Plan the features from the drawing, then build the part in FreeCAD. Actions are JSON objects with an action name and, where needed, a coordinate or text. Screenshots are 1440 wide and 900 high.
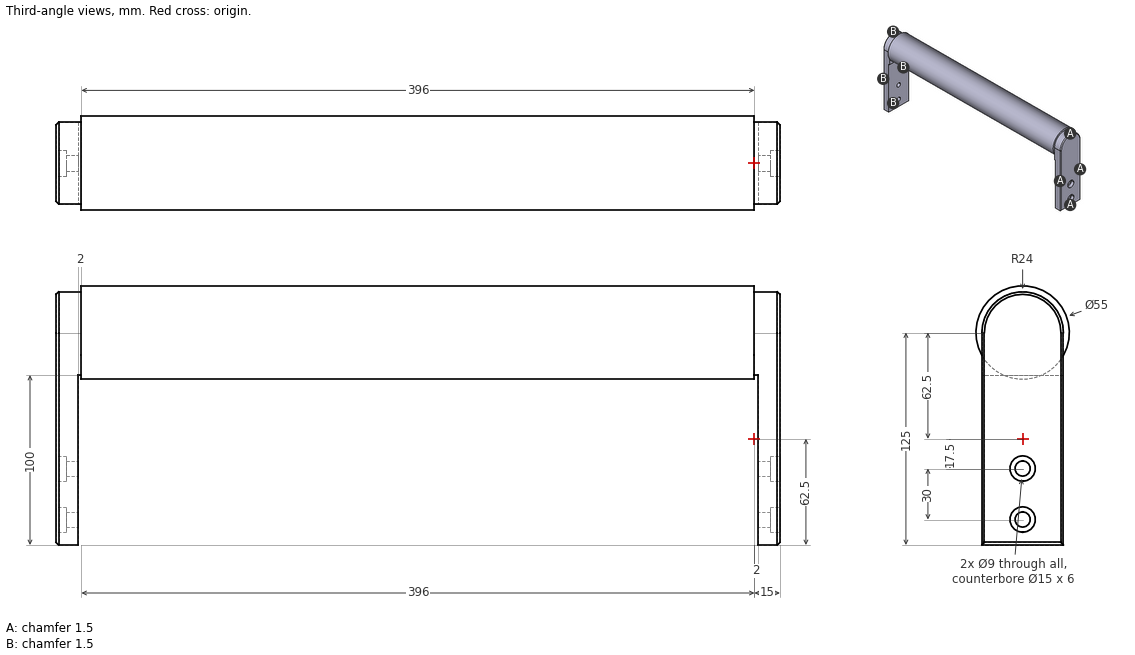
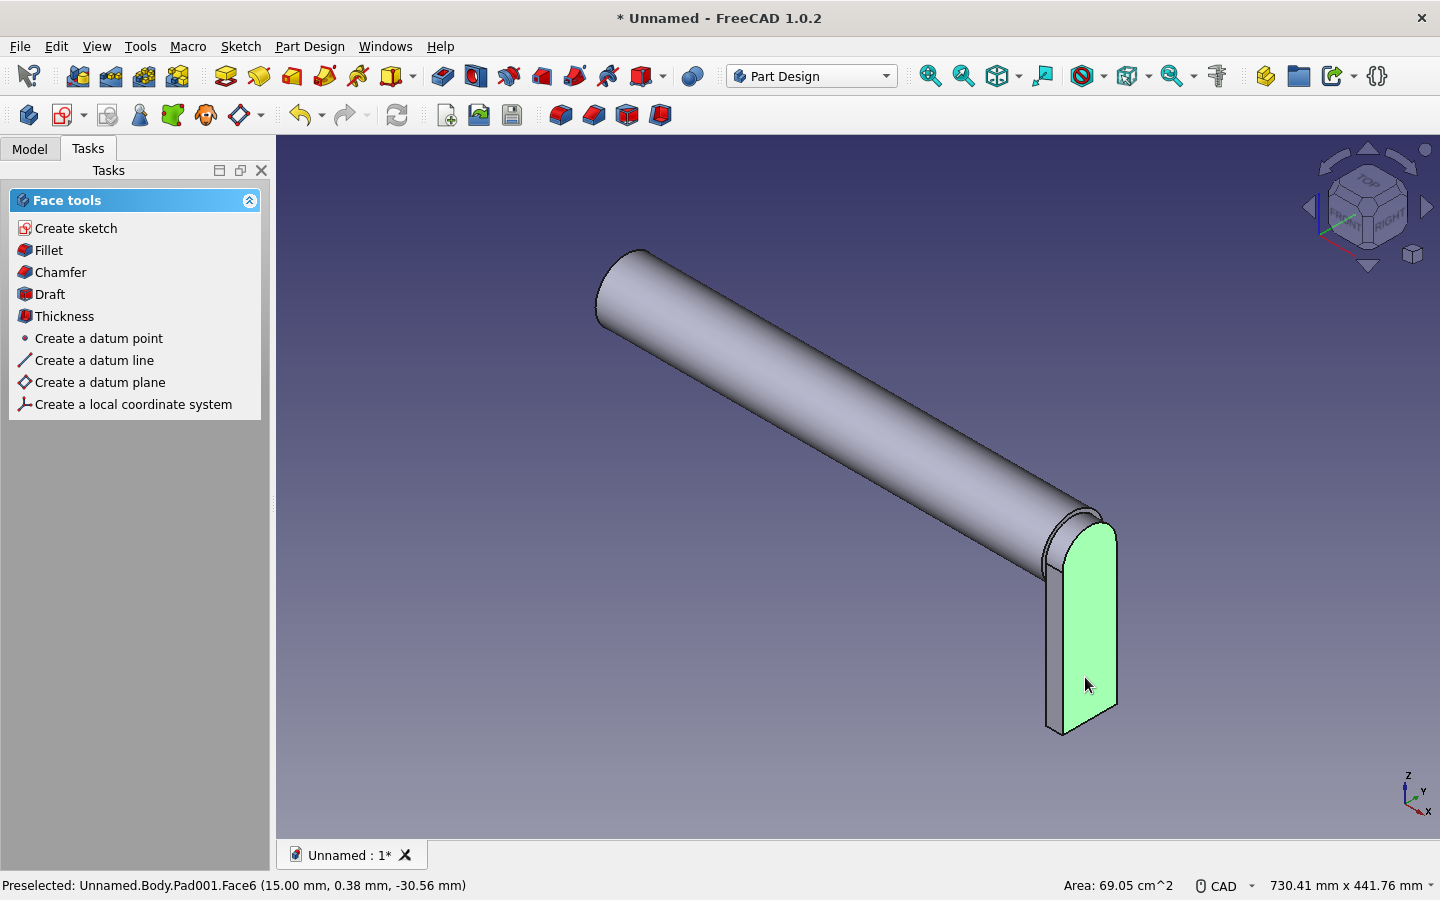
{"action": "left_click", "coordinate": [62, 116]}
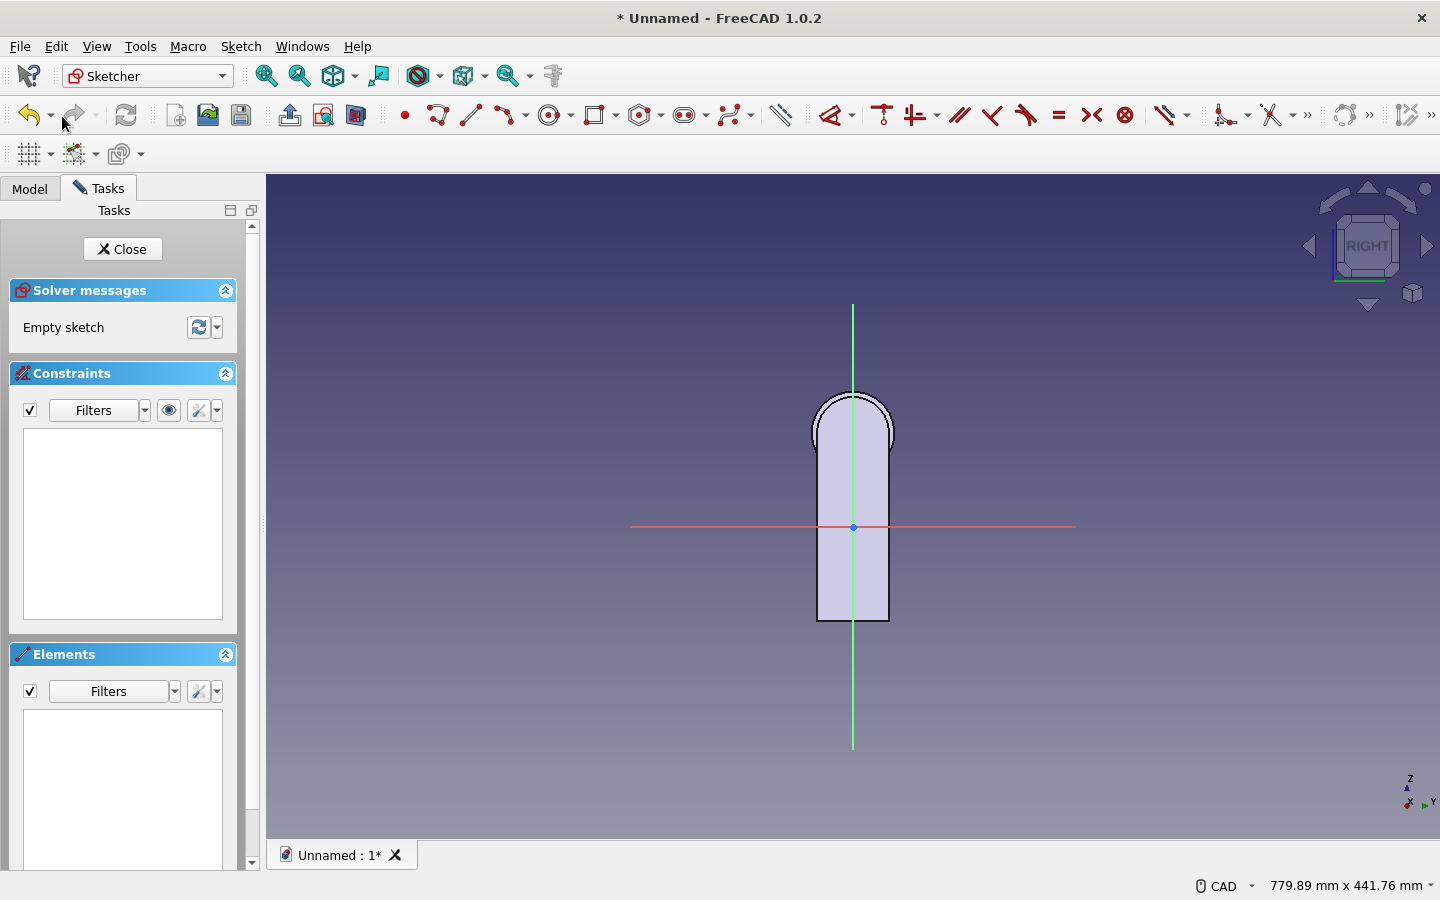
{"action": "scroll", "coordinate": [867, 578], "scroll_direction": "up", "scroll_amount": 9}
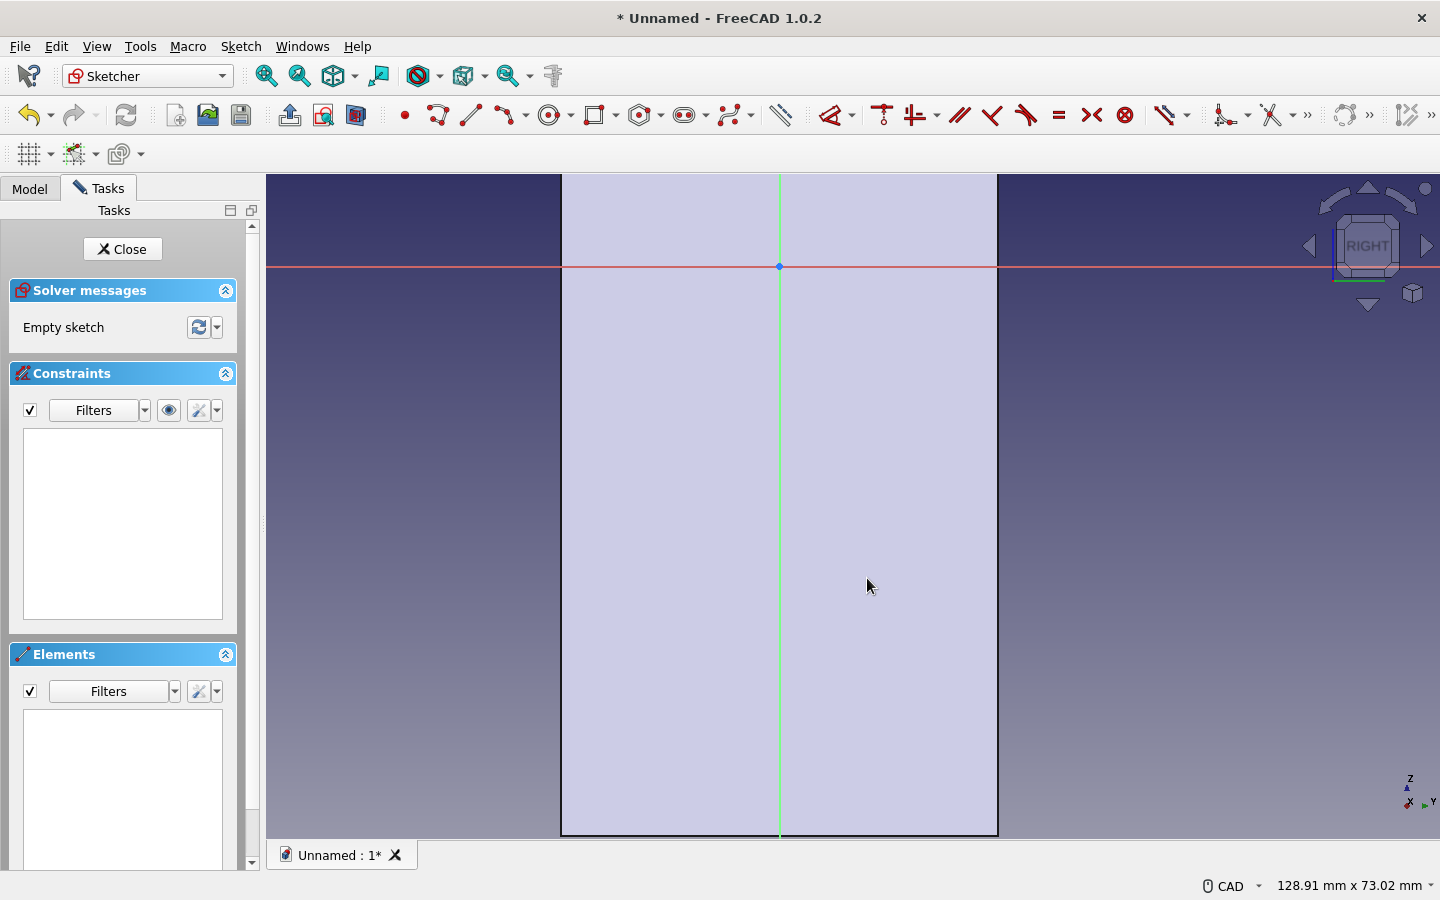
{"action": "left_click", "coordinate": [548, 116]}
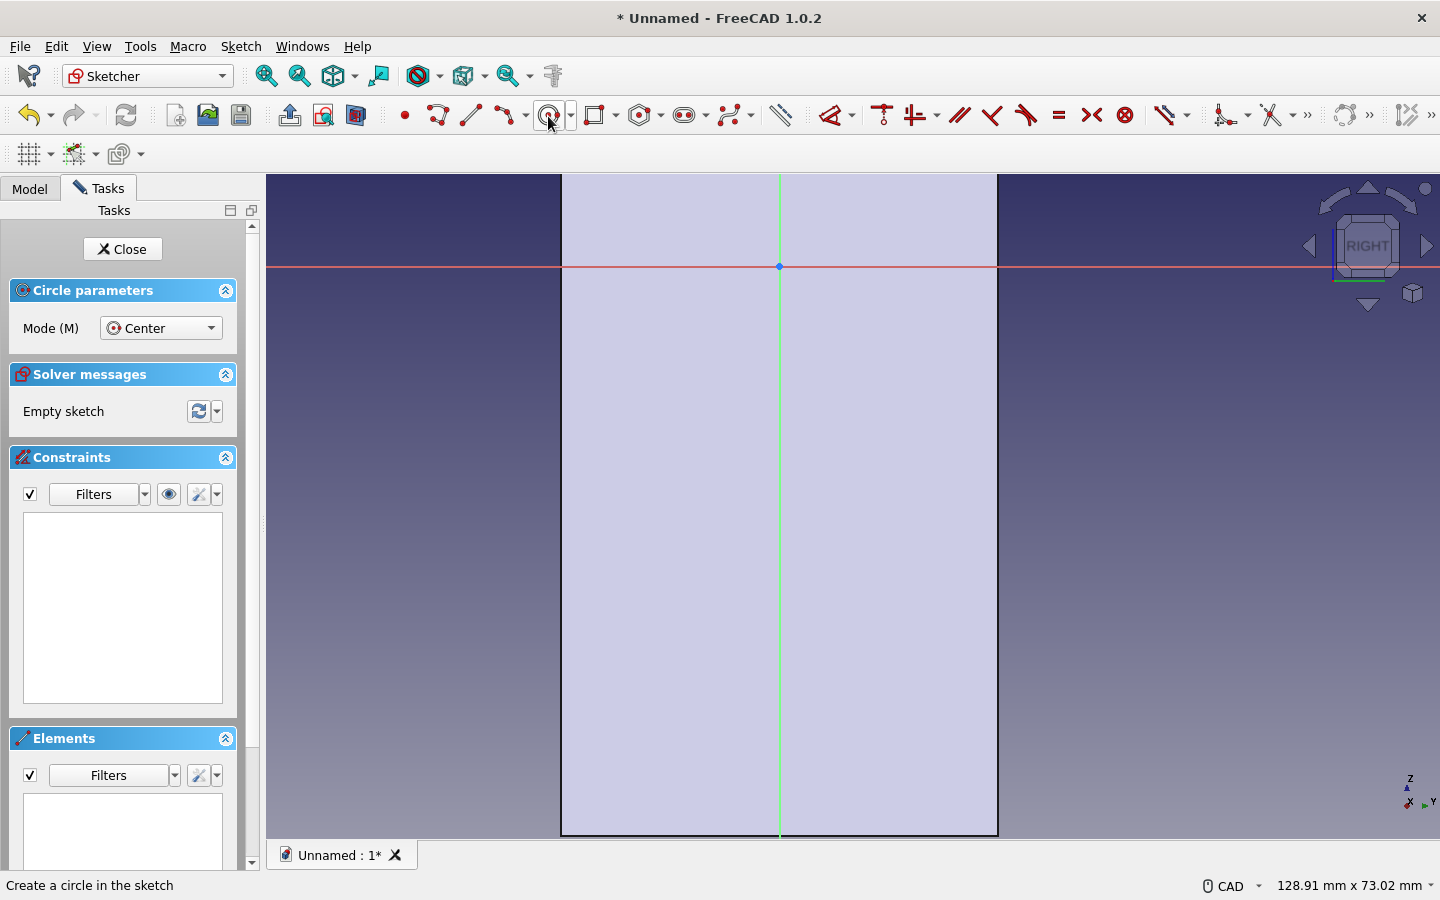
{"action": "left_click", "coordinate": [780, 426]}
{"action": "mouse_move", "coordinate": [809, 397]}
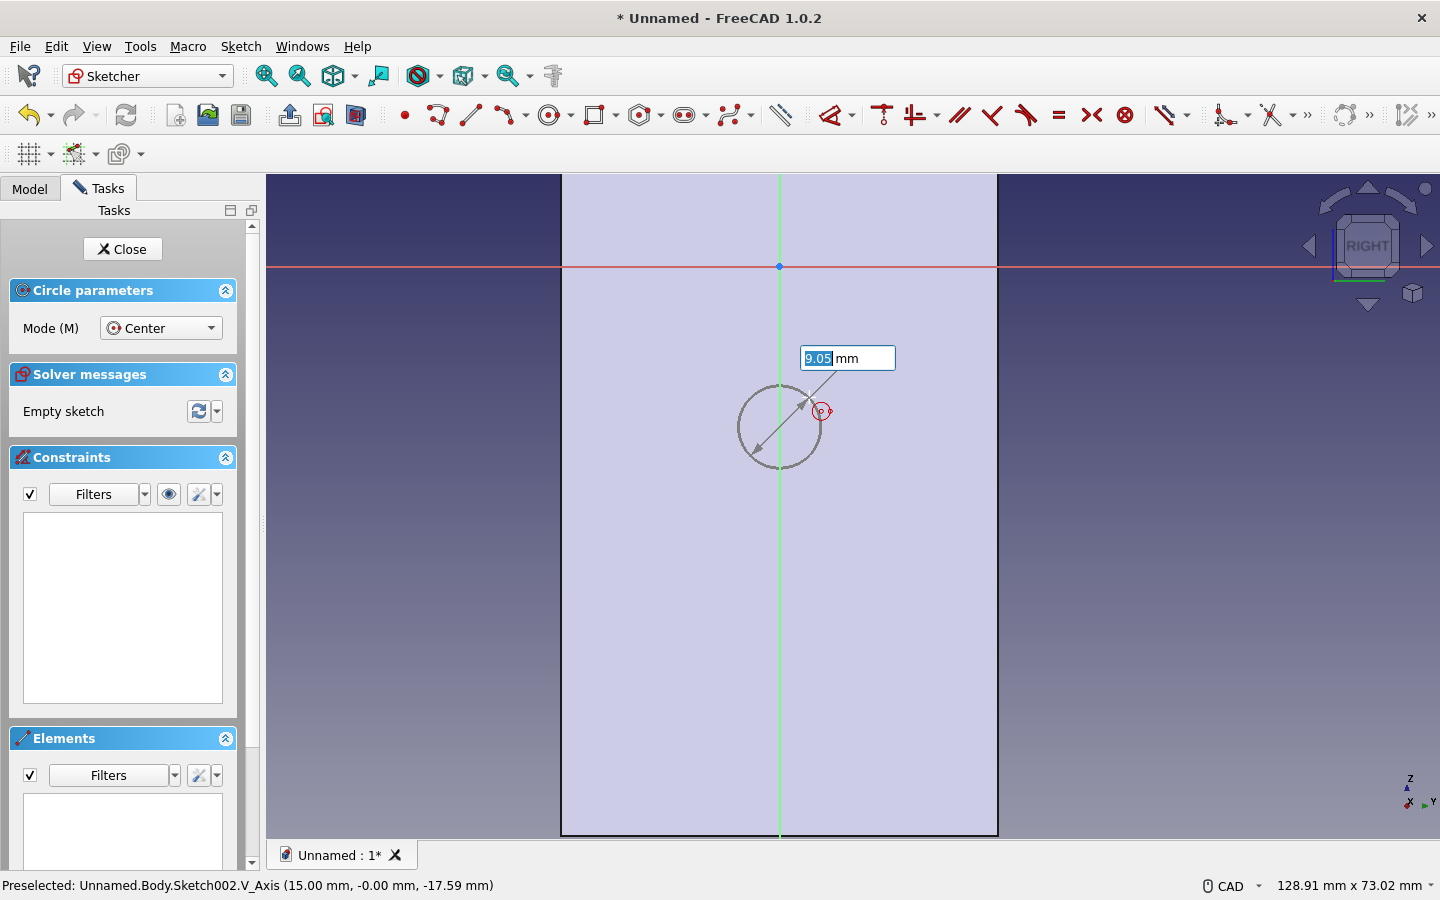
{"action": "type", "text": "9"}
{"action": "key", "text": "Return"}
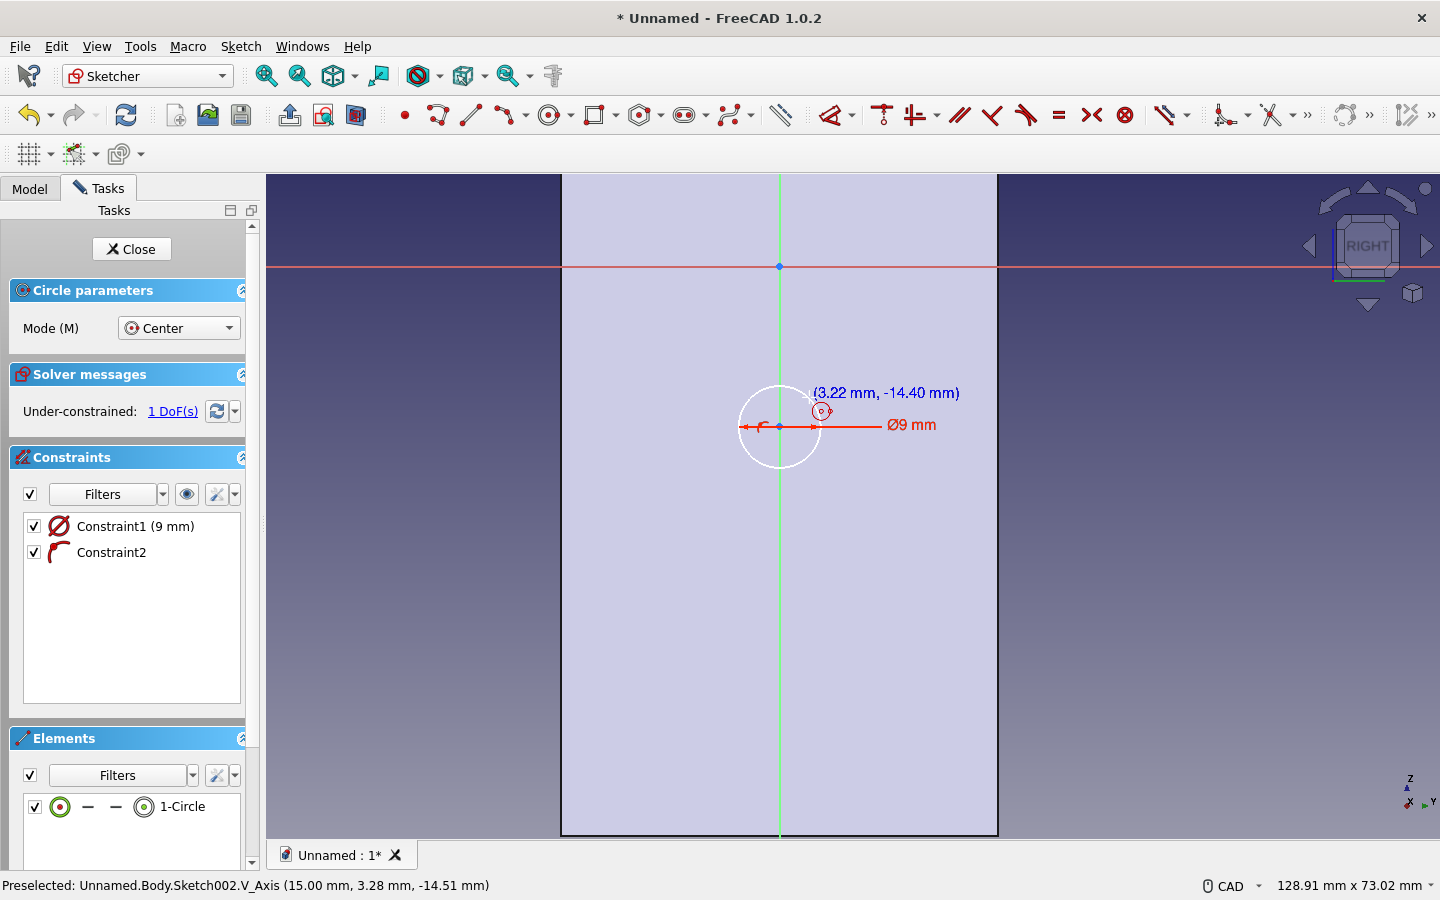
{"action": "left_click", "coordinate": [780, 699]}
{"action": "mouse_move", "coordinate": [809, 670]}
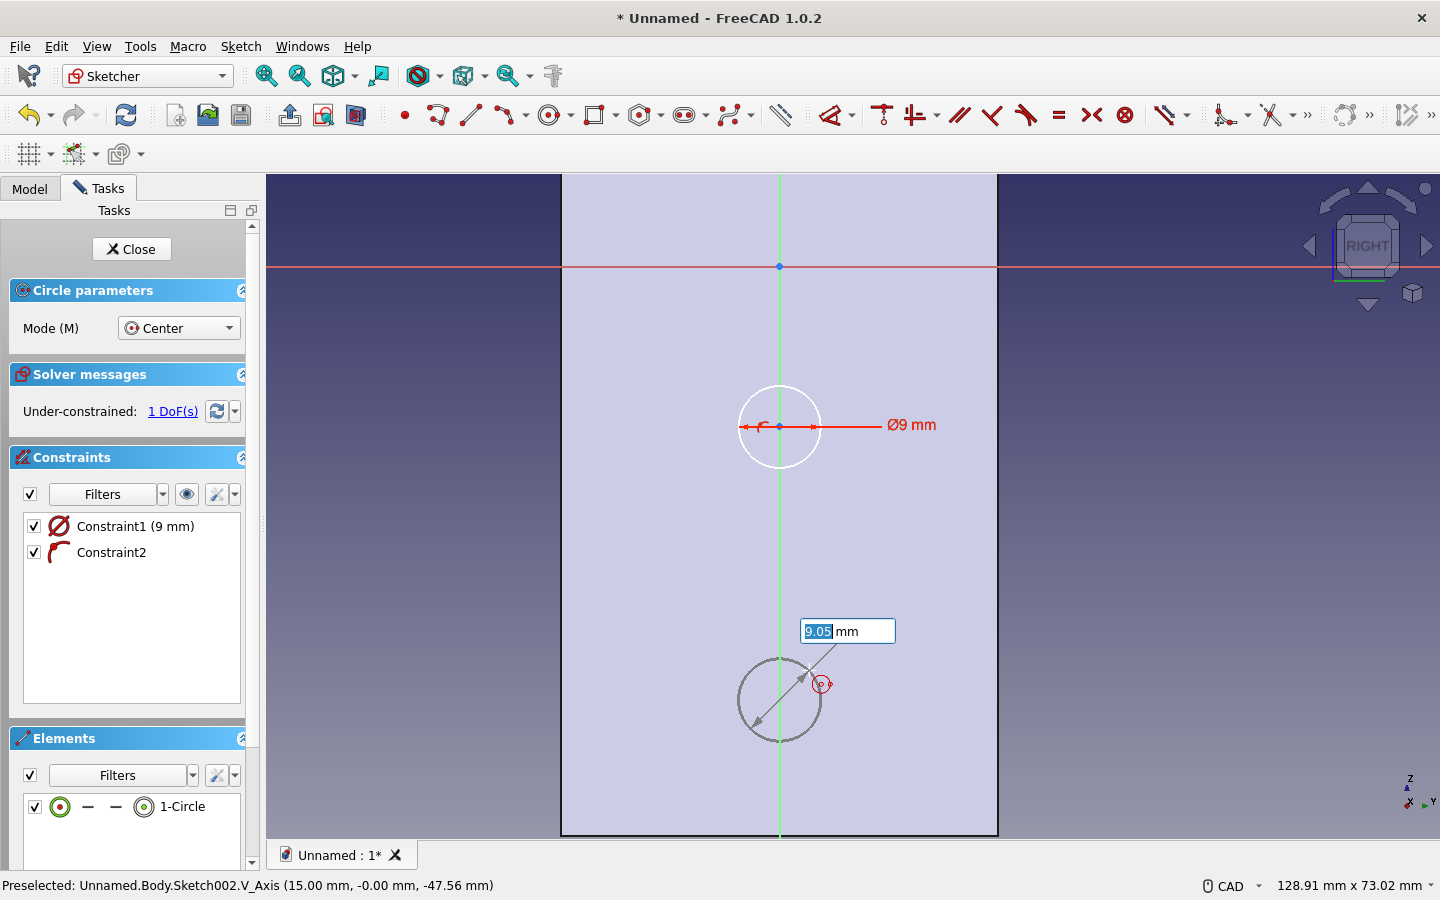
{"action": "type", "text": "9"}
{"action": "key", "text": "Return"}
{"action": "key", "text": "Escape"}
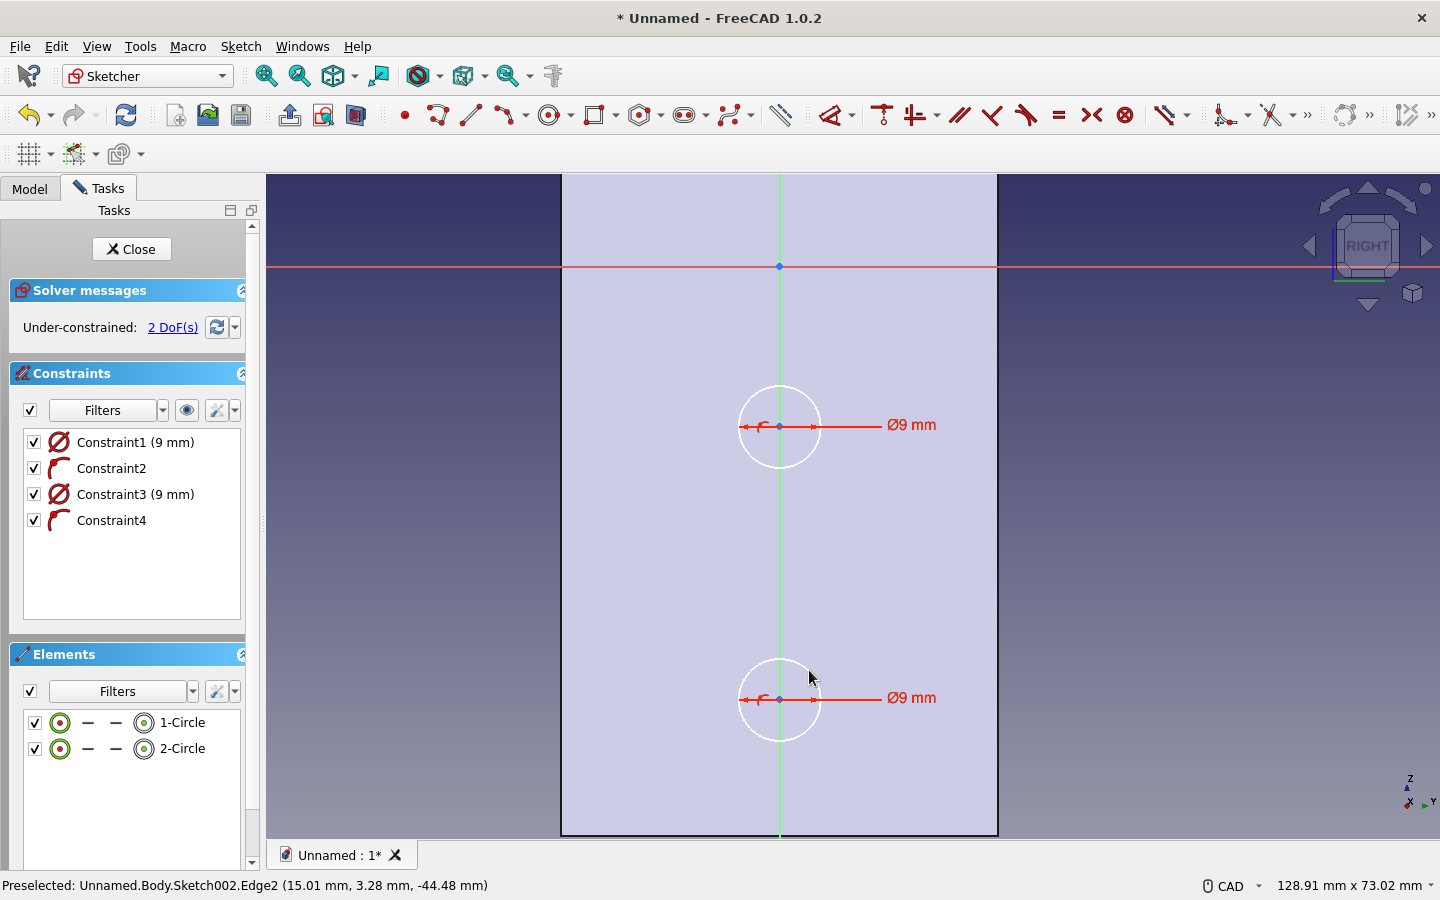
{"action": "left_click", "coordinate": [830, 116]}